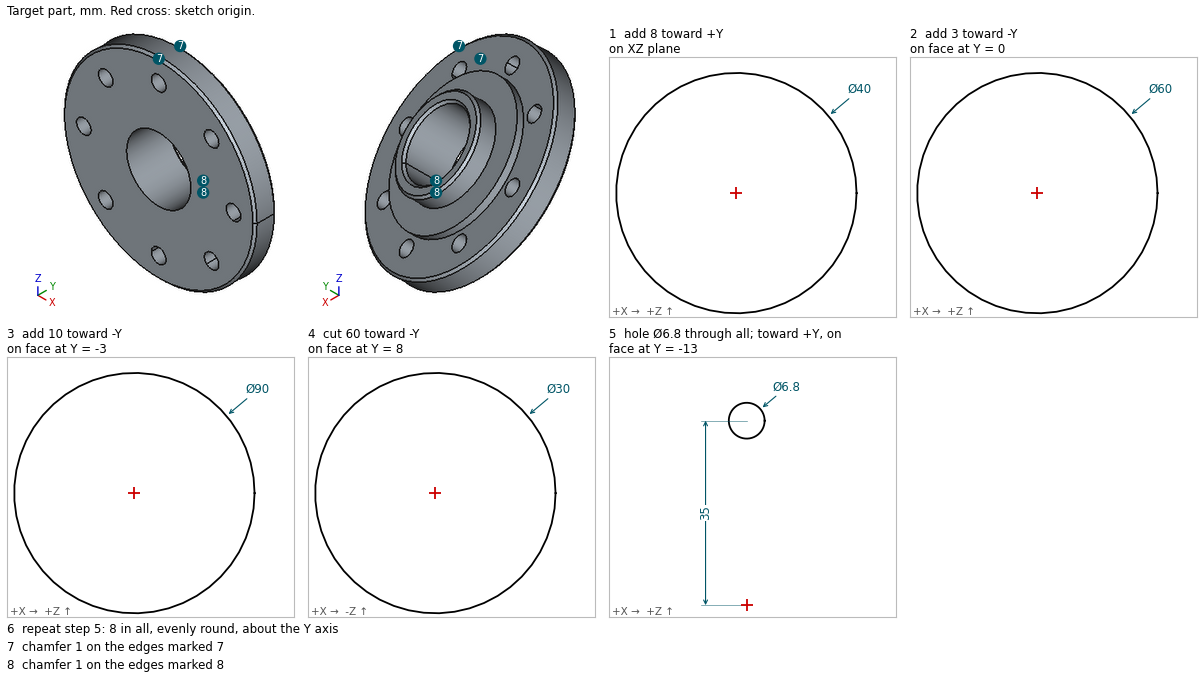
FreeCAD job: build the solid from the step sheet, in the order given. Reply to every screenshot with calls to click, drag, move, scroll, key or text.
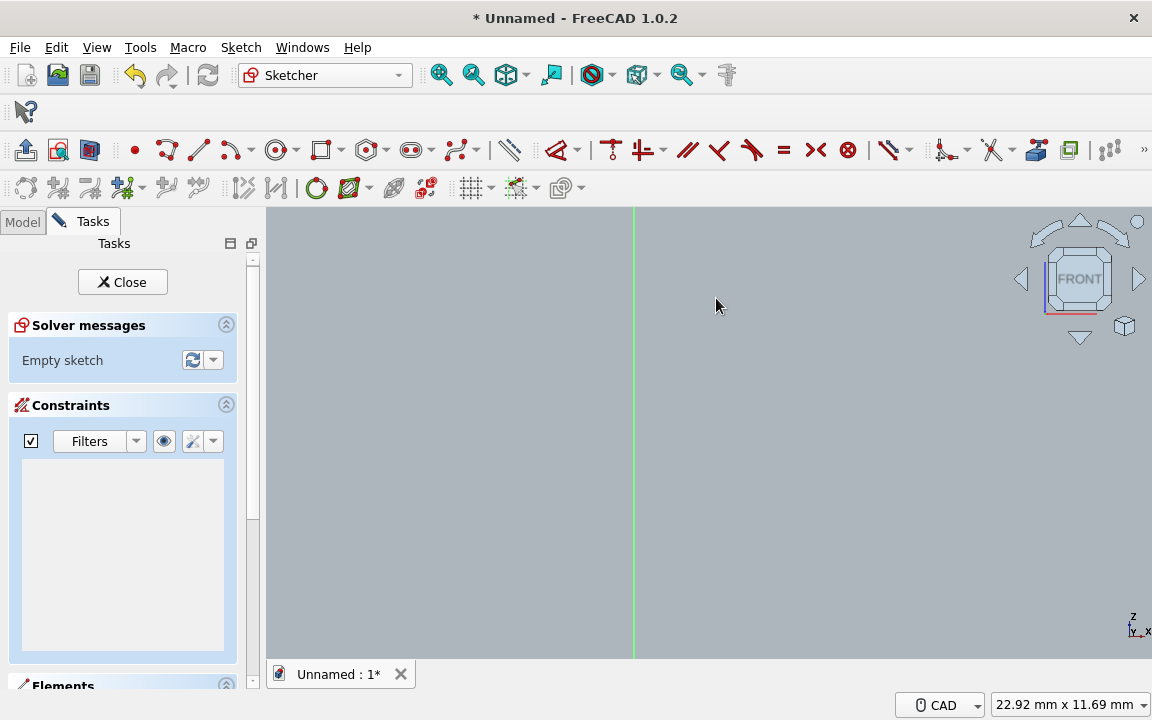
click(276, 150)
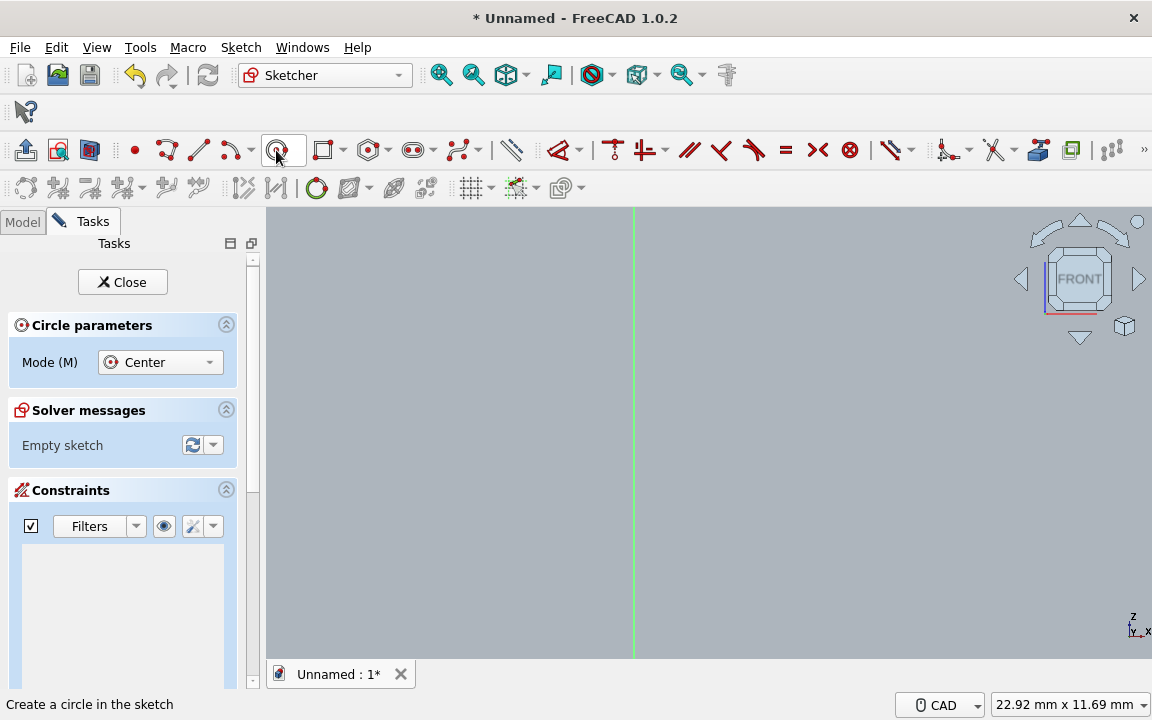
click(634, 431)
move(727, 338)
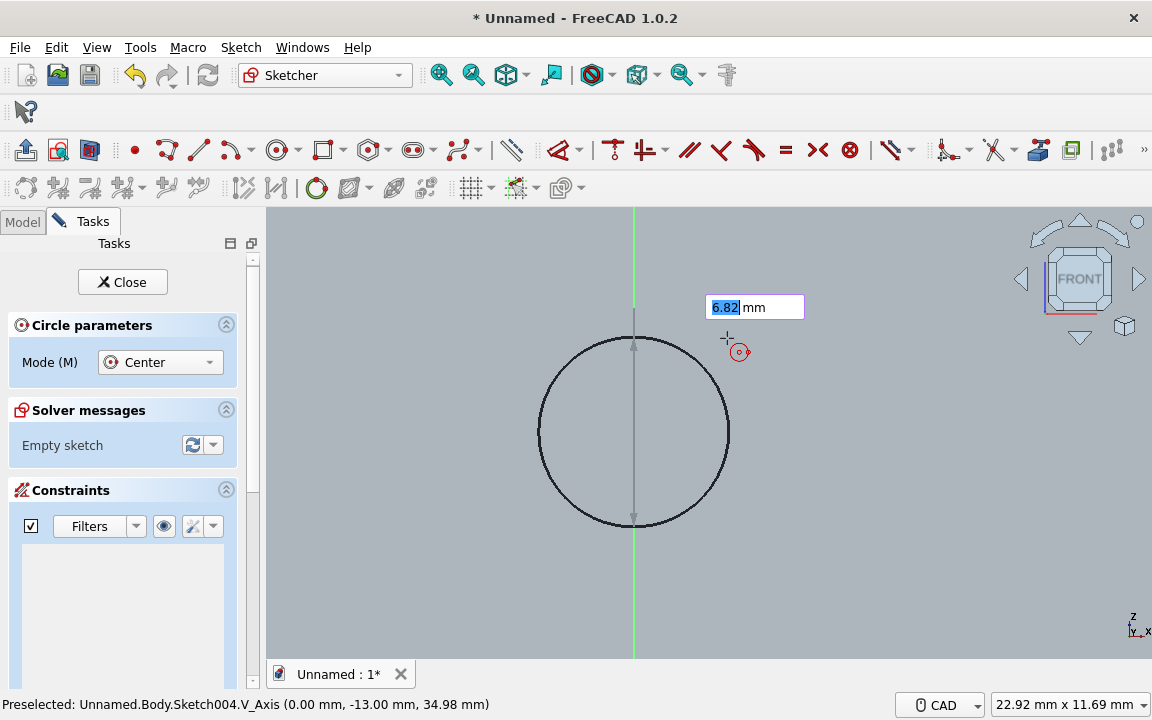
text(6.8)
key(Return)
key(Escape)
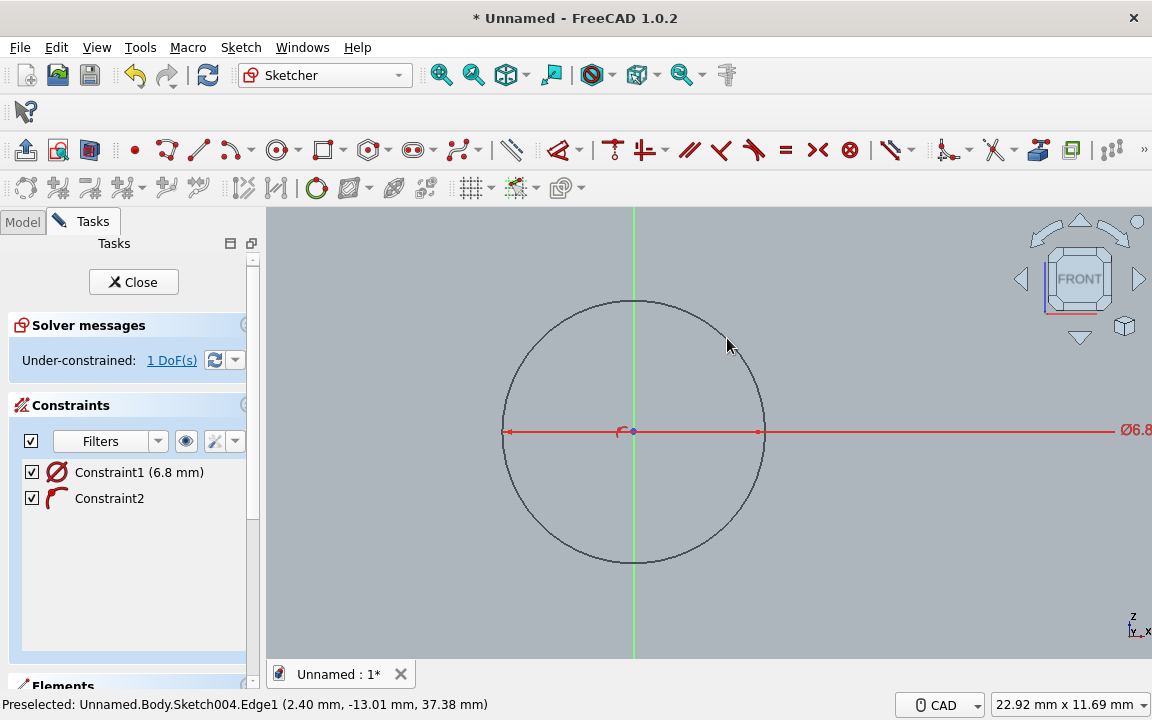
click(558, 150)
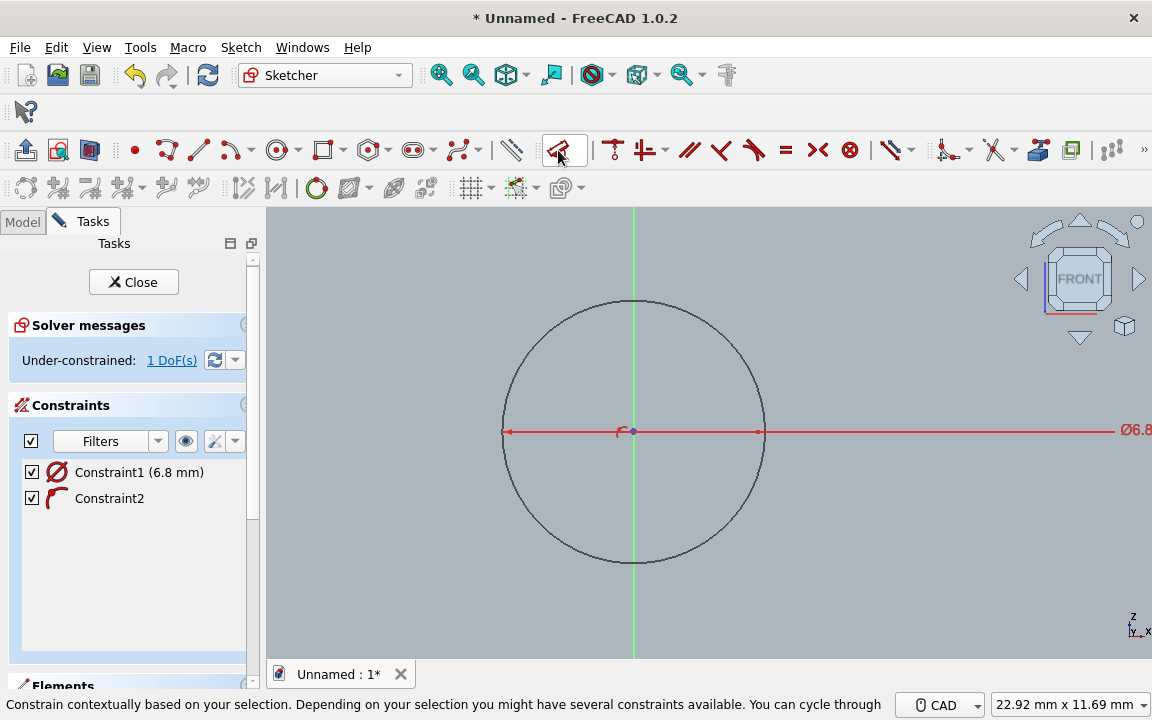
click(634, 432)
click(668, 532)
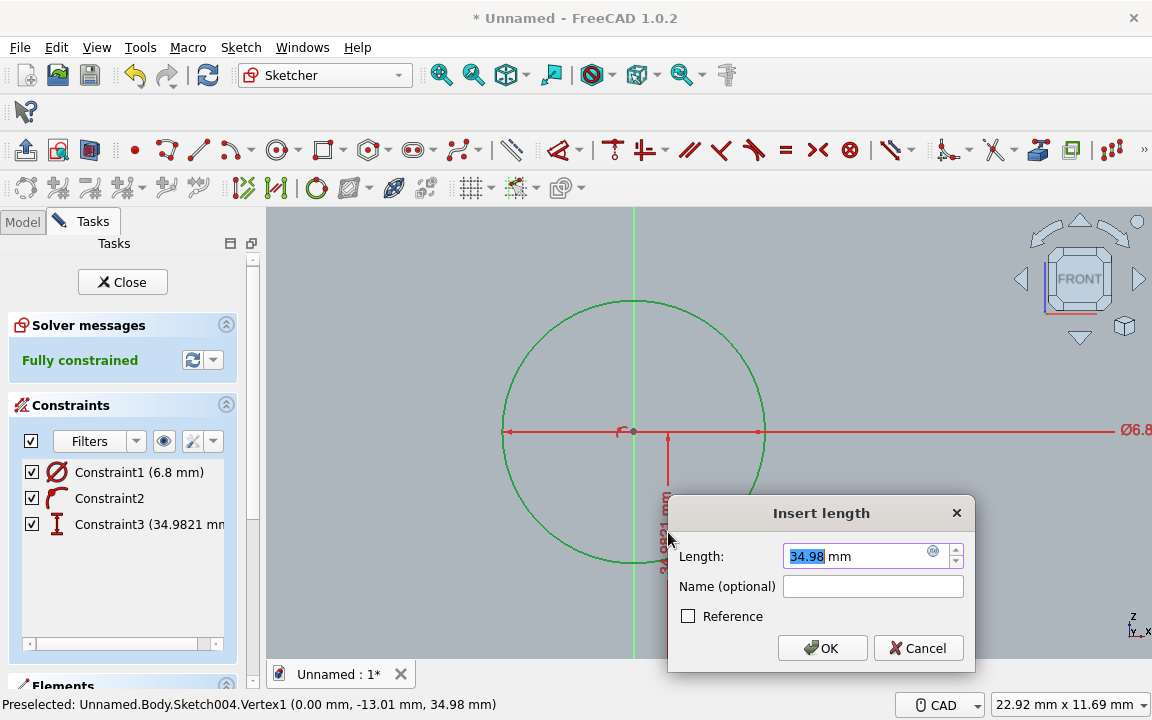
text(35)
key(Return)
key(Escape)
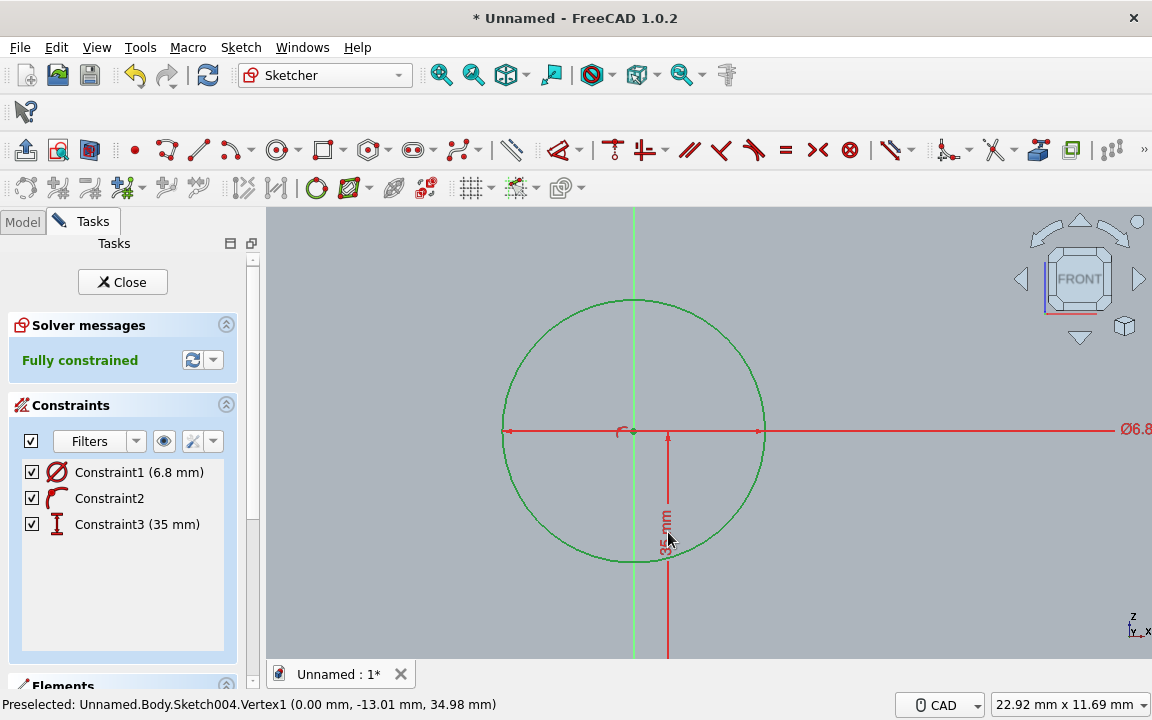
click(123, 282)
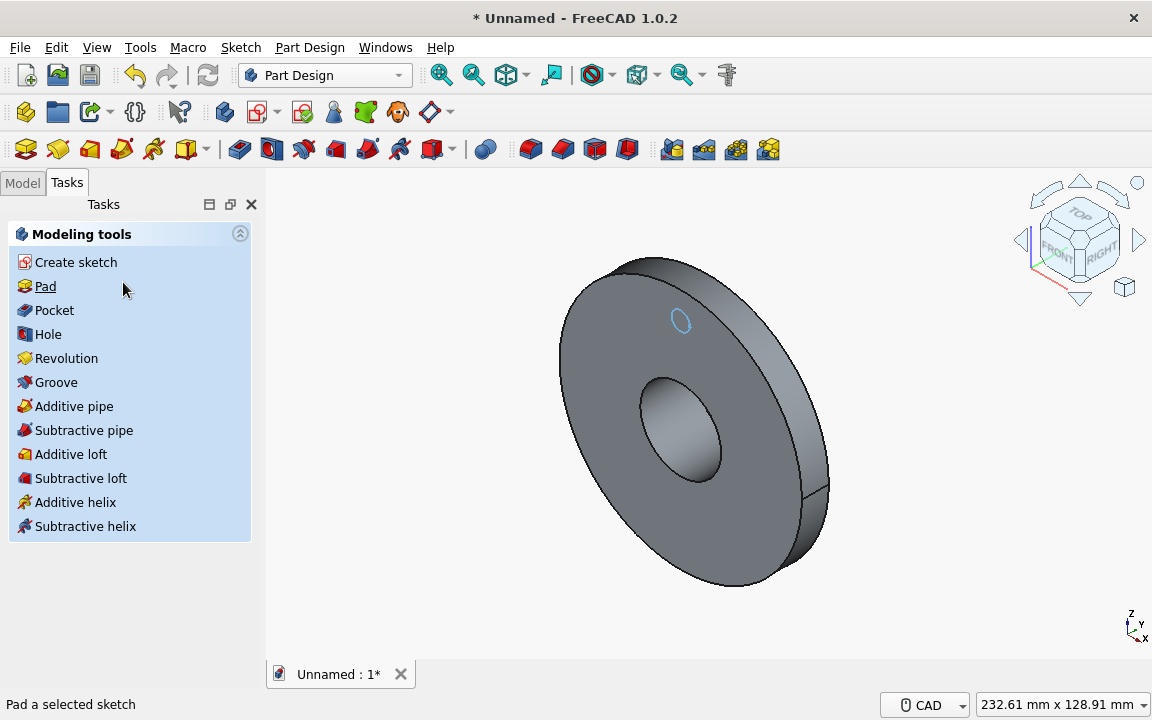
click(272, 150)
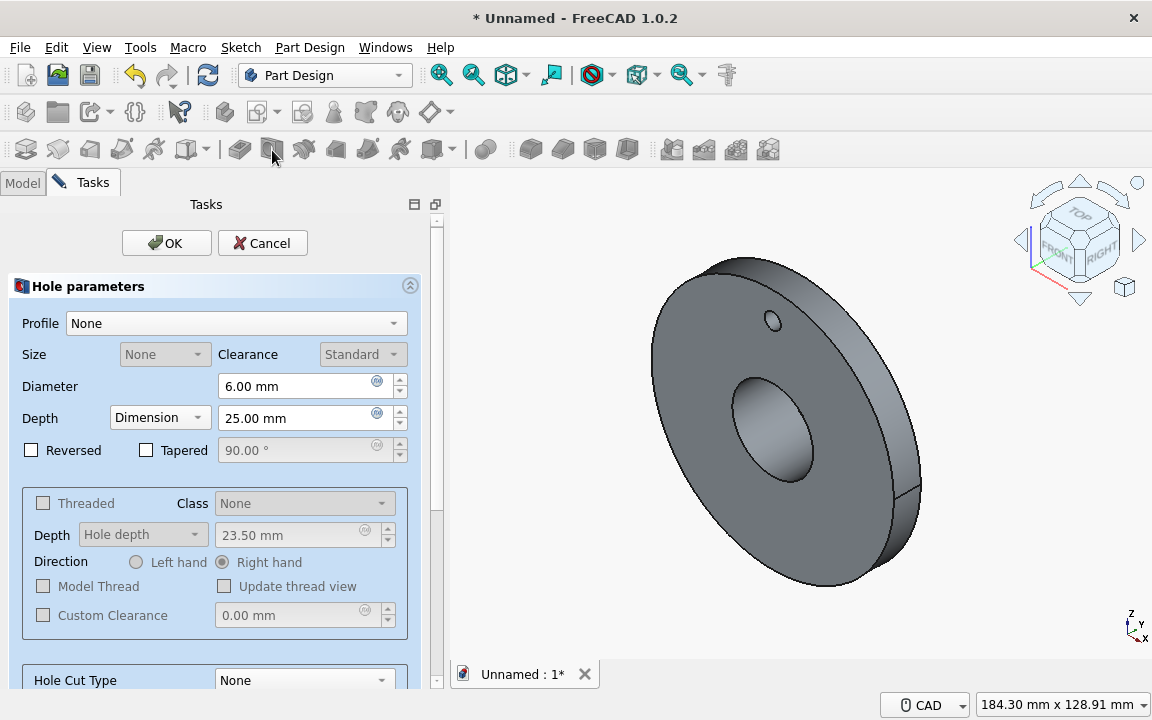
triple_click(305, 386)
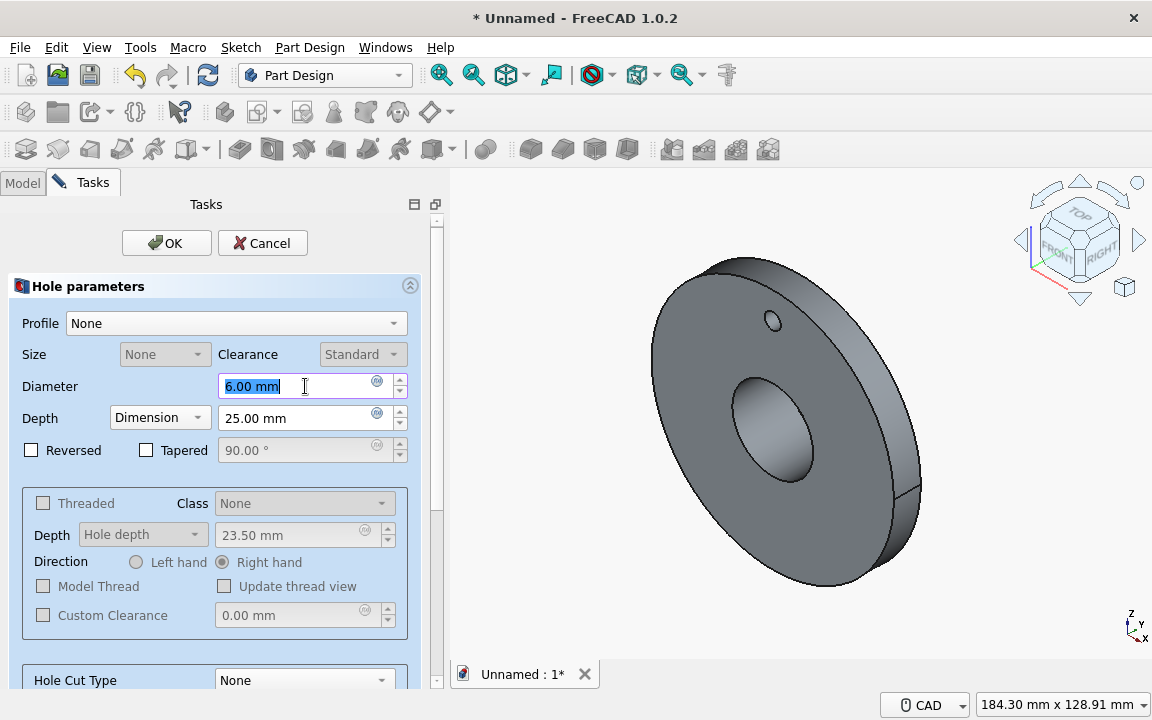
text(6.8)
key(Tab)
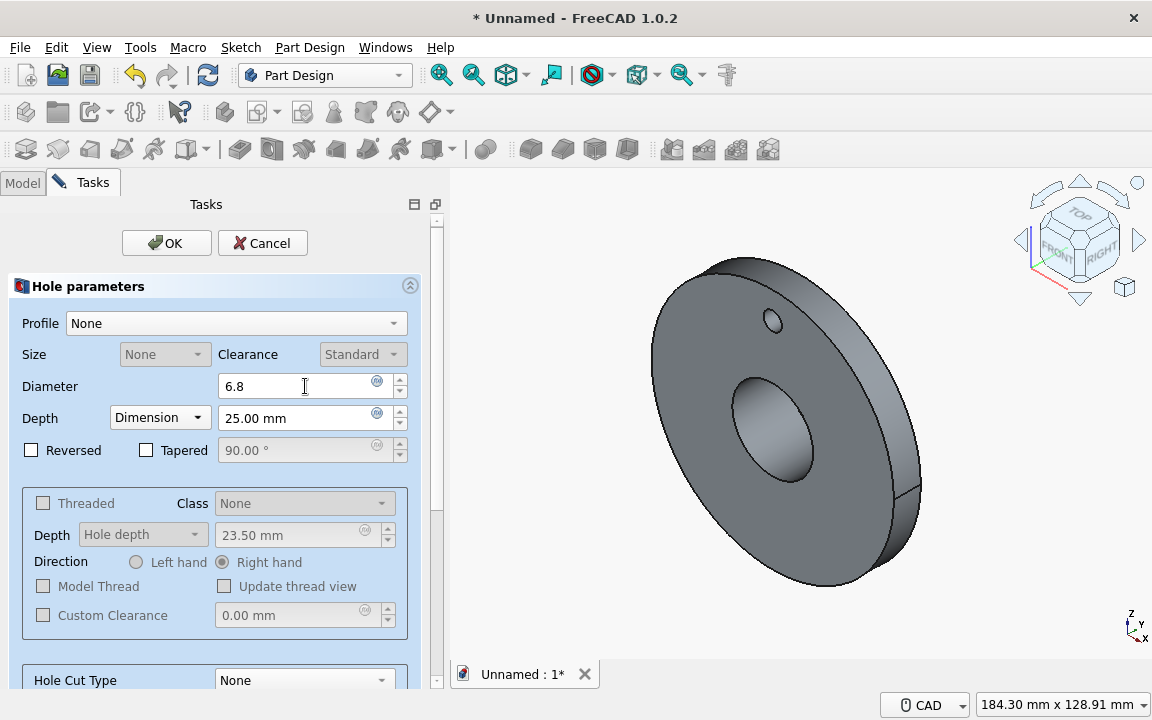
click(161, 418)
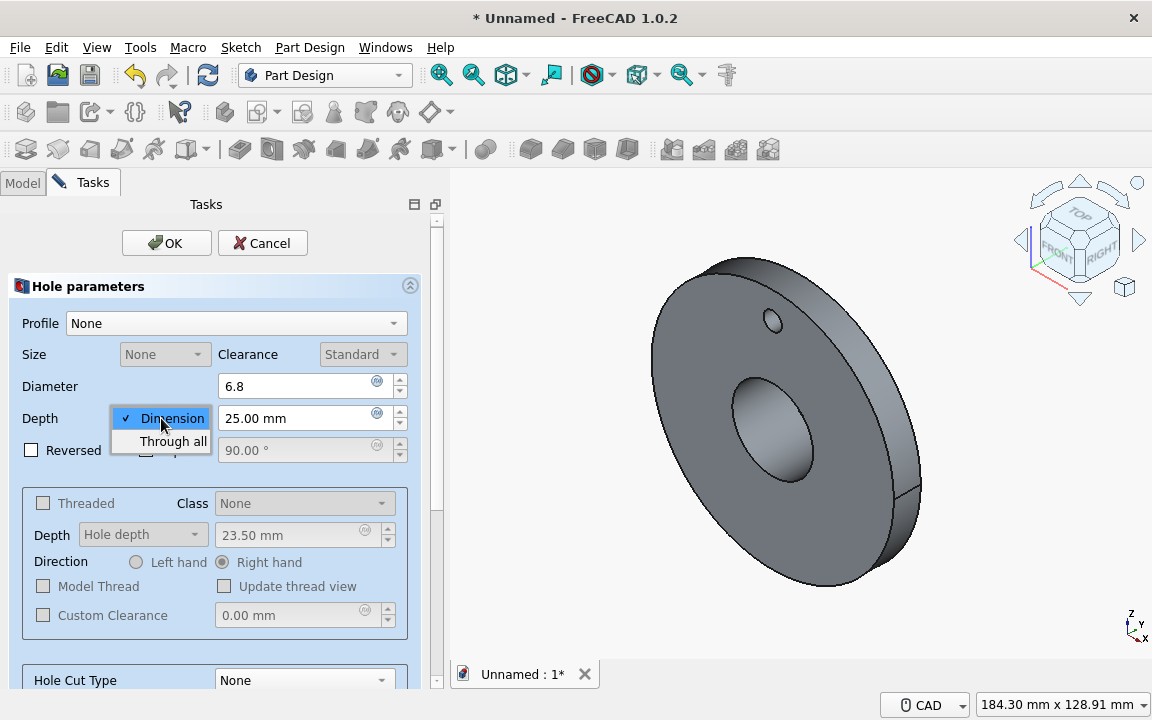
click(160, 442)